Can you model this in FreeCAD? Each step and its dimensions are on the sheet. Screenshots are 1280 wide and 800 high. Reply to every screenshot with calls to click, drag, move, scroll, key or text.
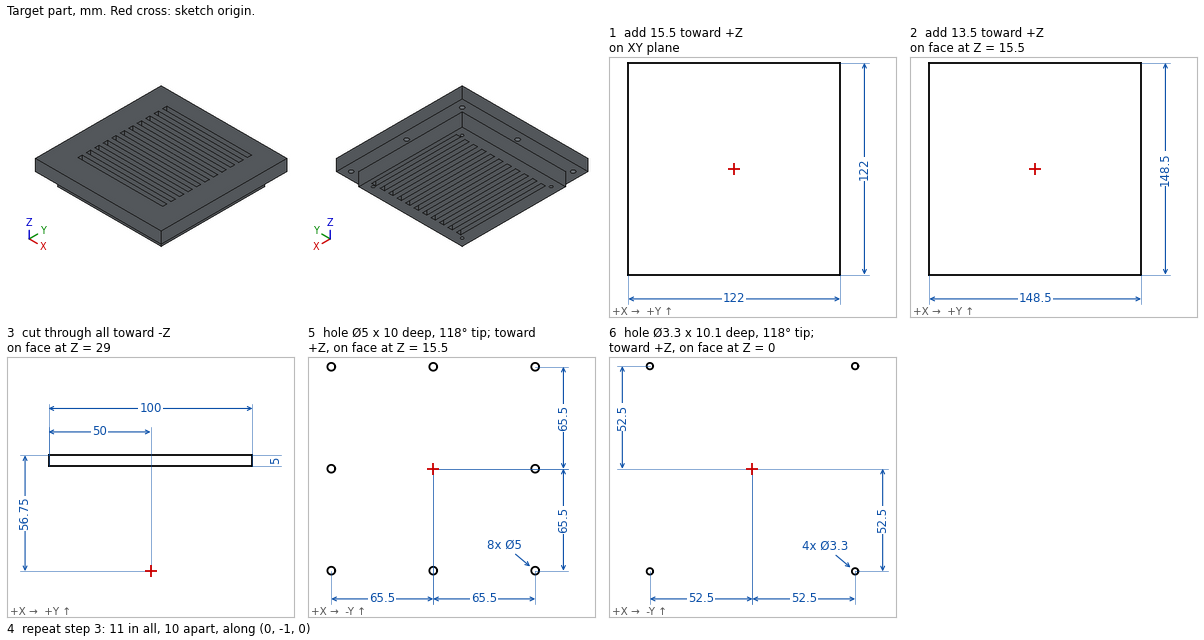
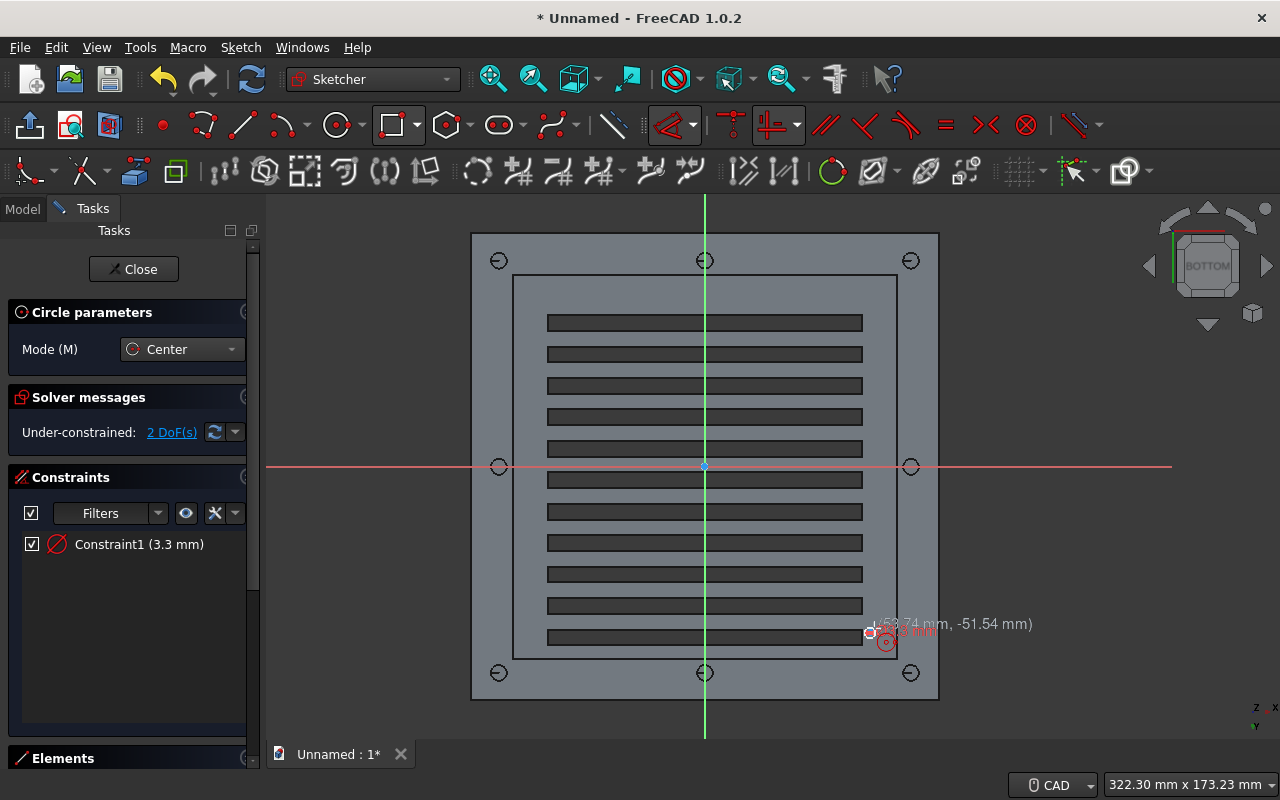
scroll(540, 632, up, 8)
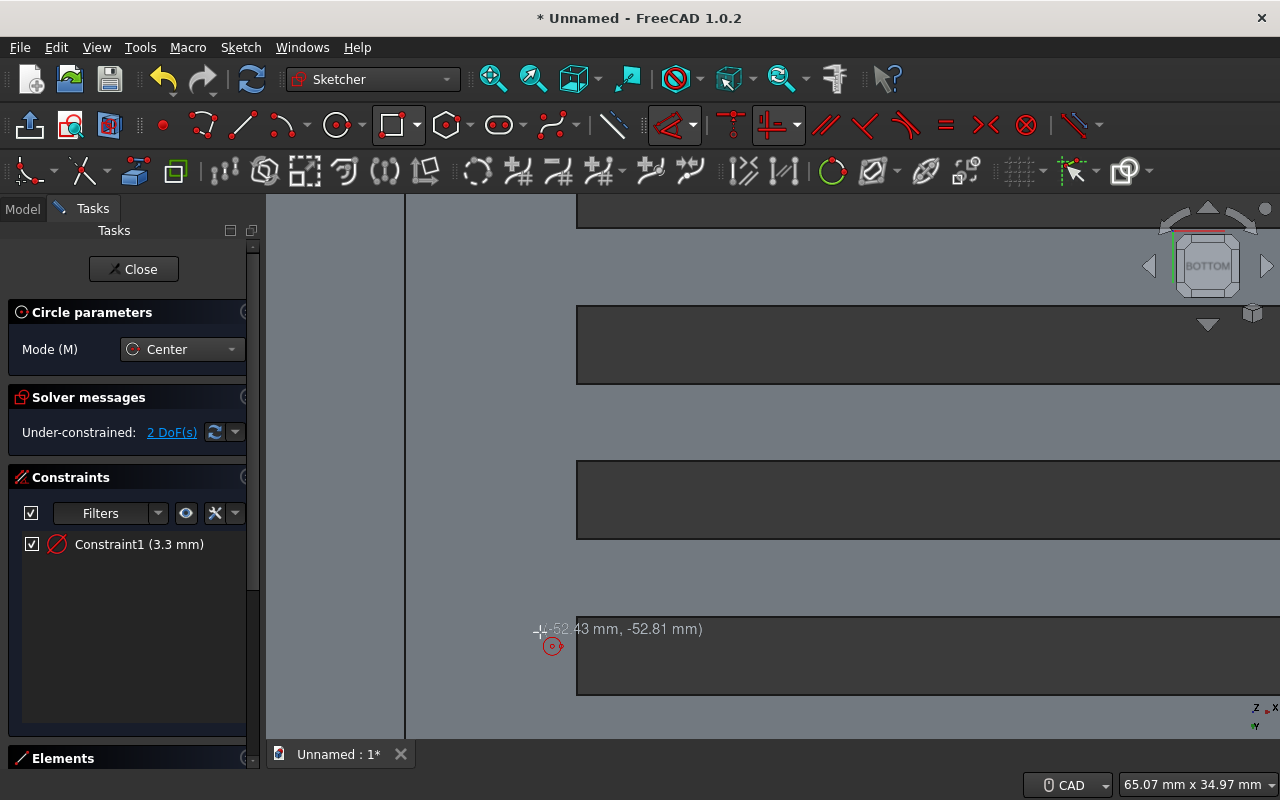
scroll(540, 632, down, 8)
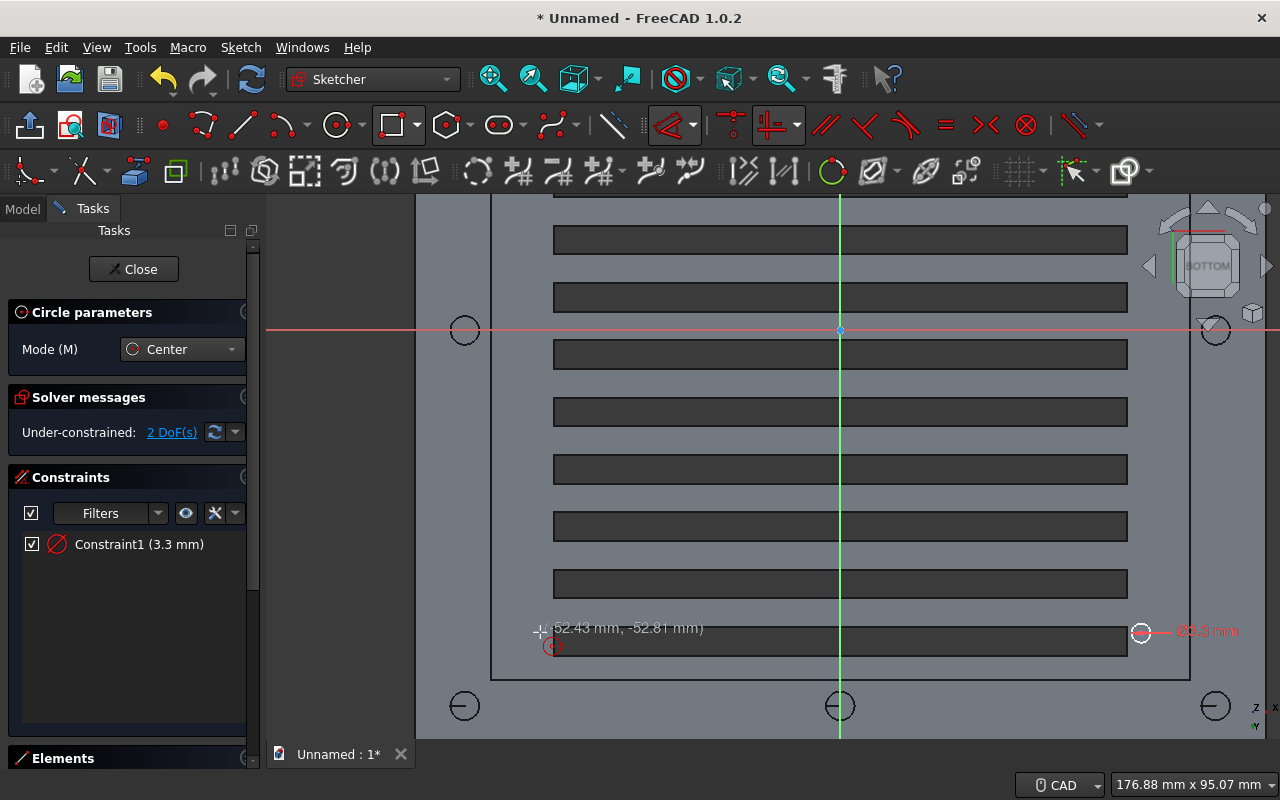
click(540, 632)
move(543, 628)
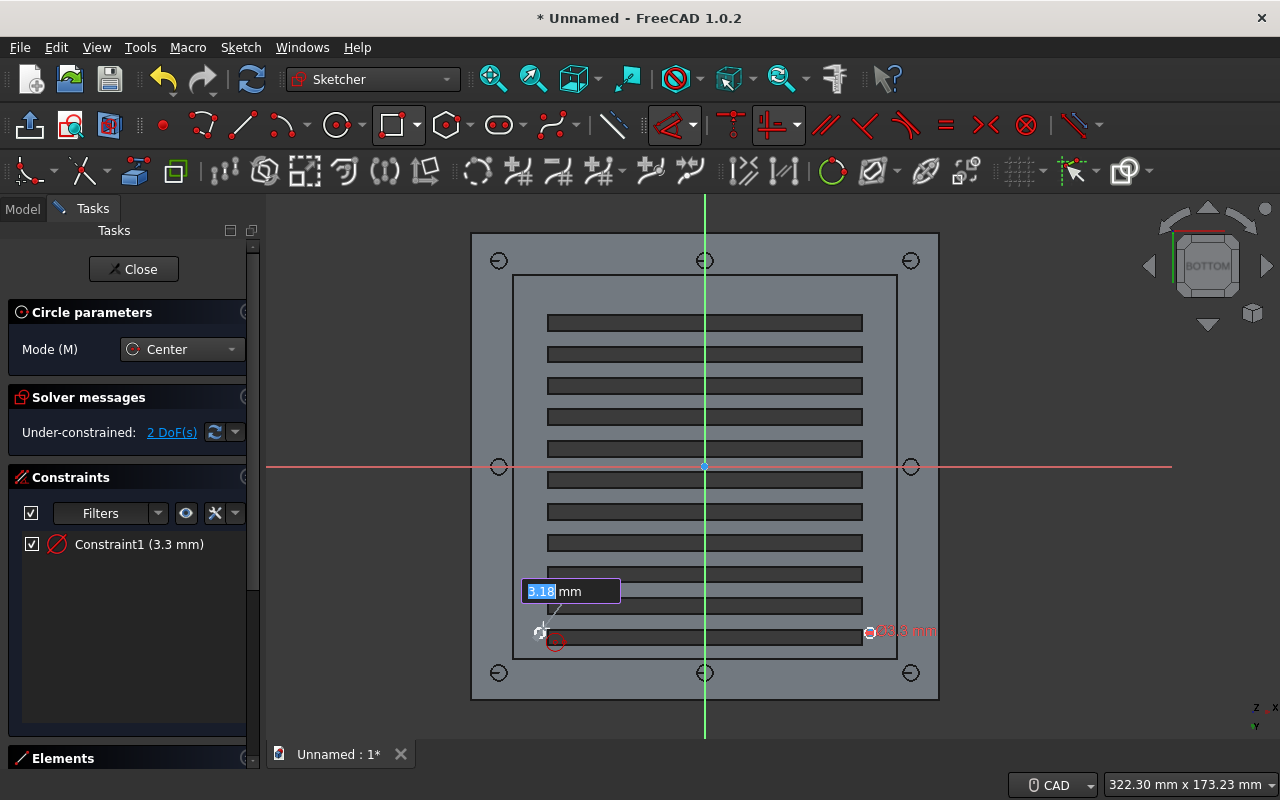
text(3.3)
key(Return)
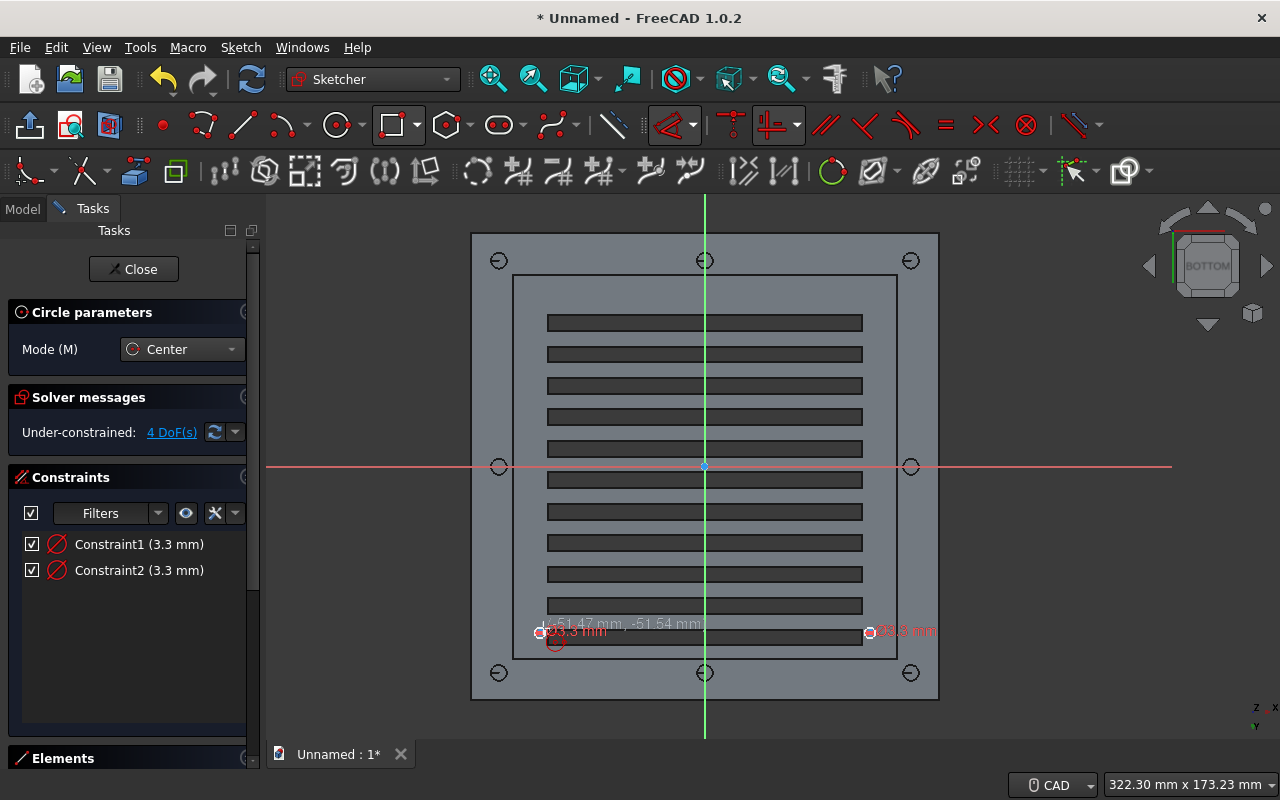
scroll(540, 302, up, 8)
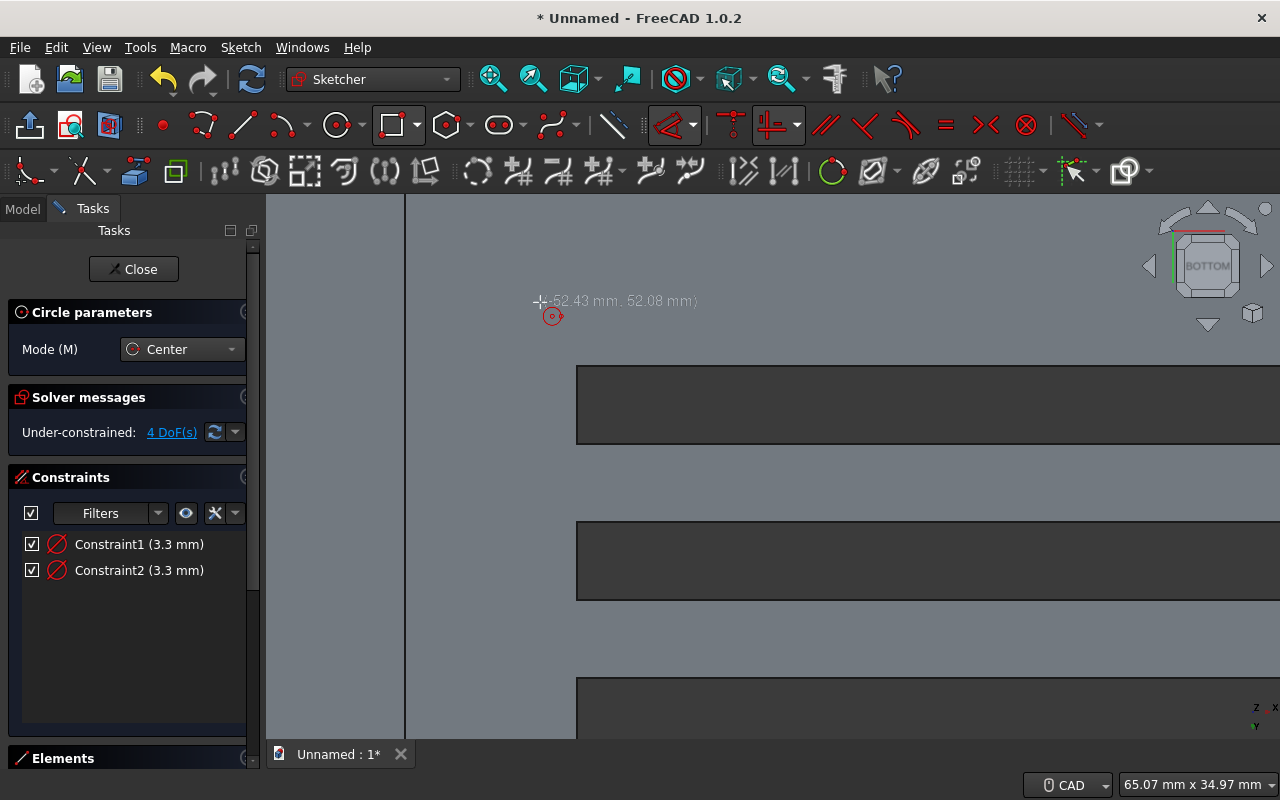
scroll(540, 302, down, 8)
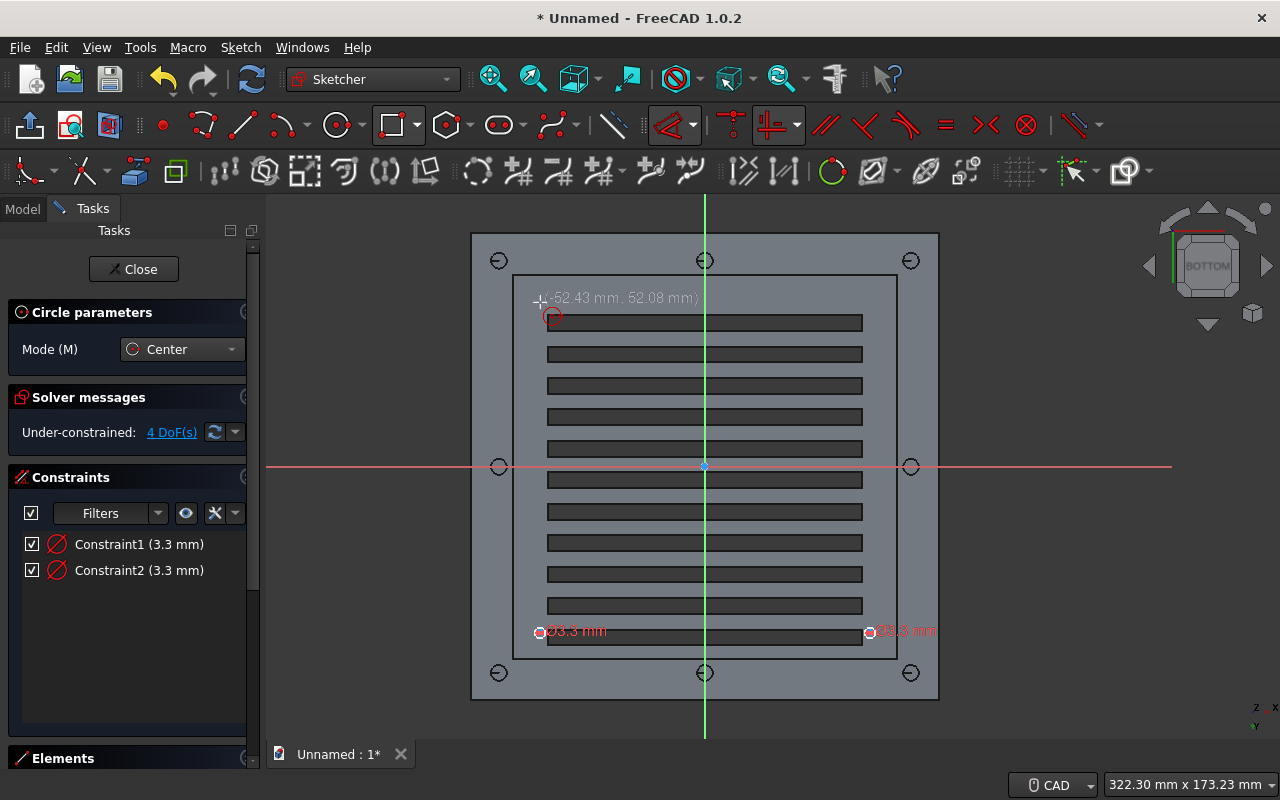
click(540, 302)
move(543, 298)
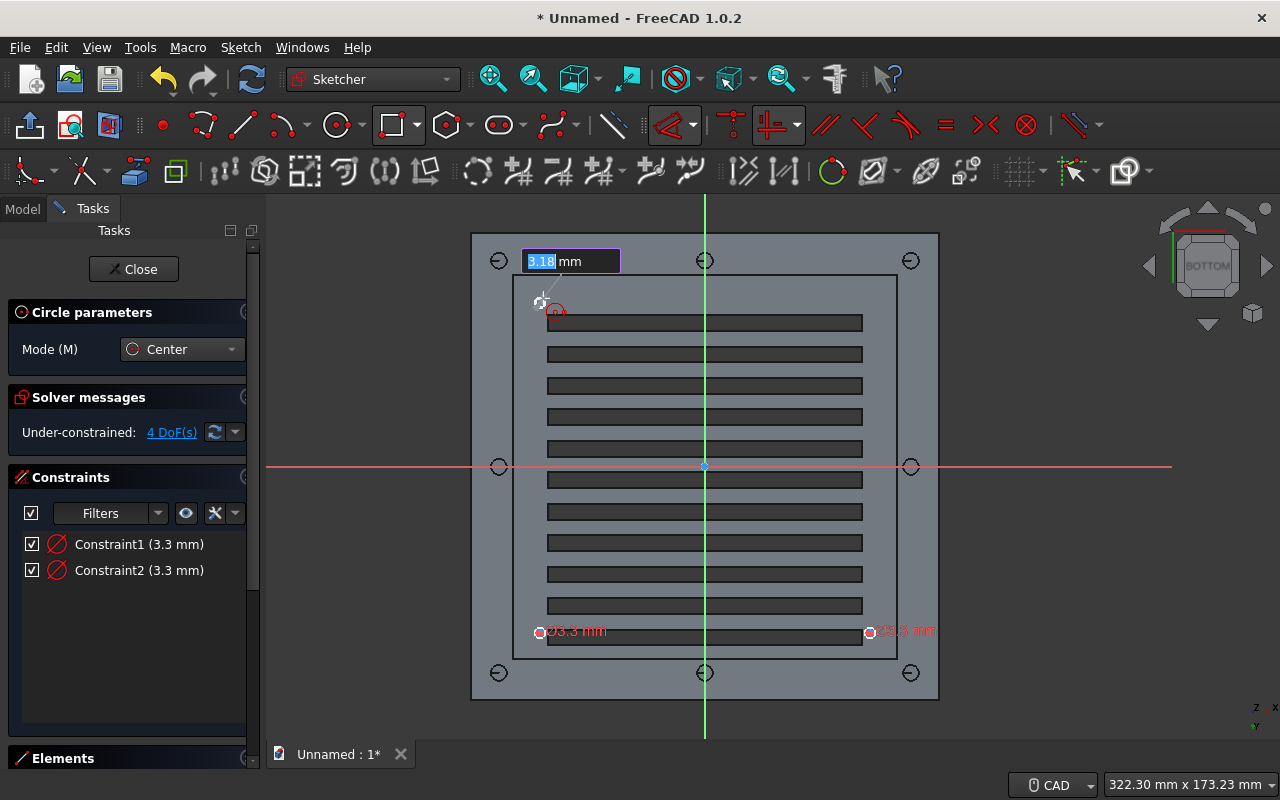
text(3.3)
key(Return)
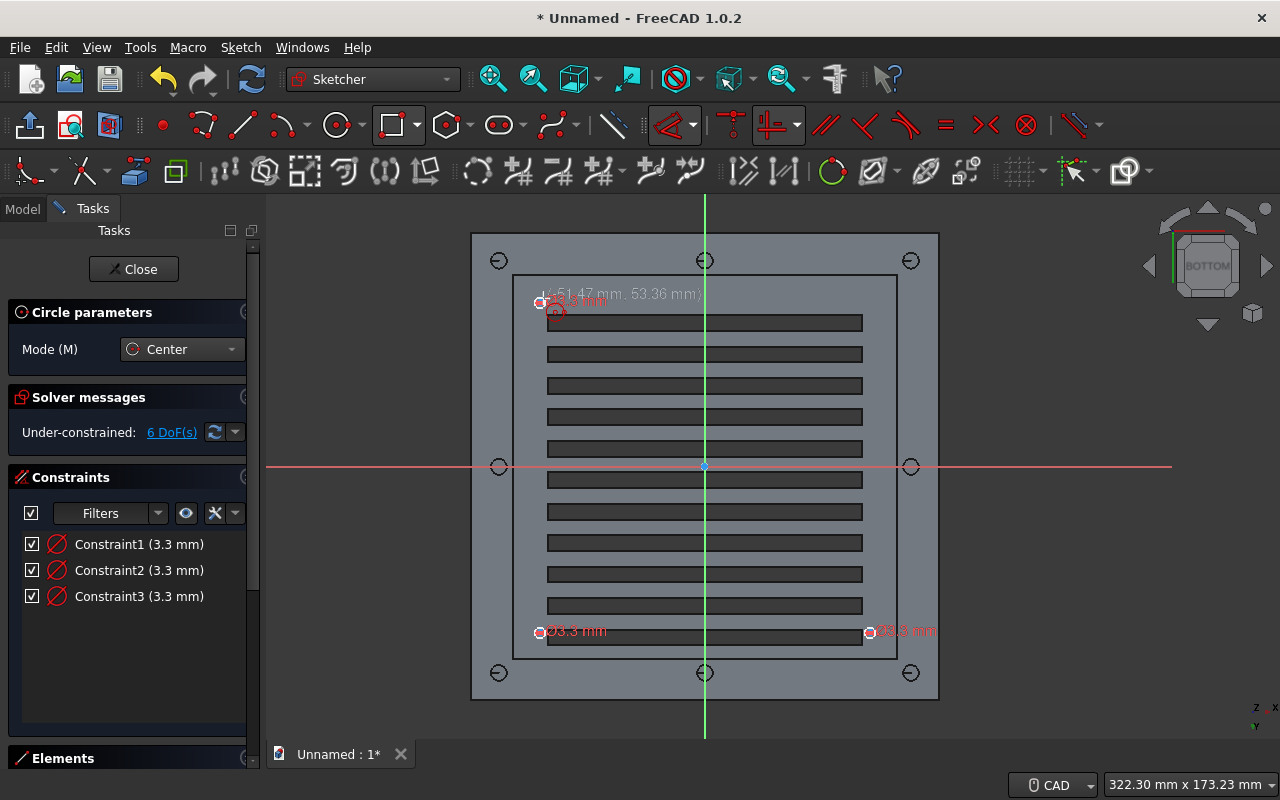
scroll(870, 302, up, 8)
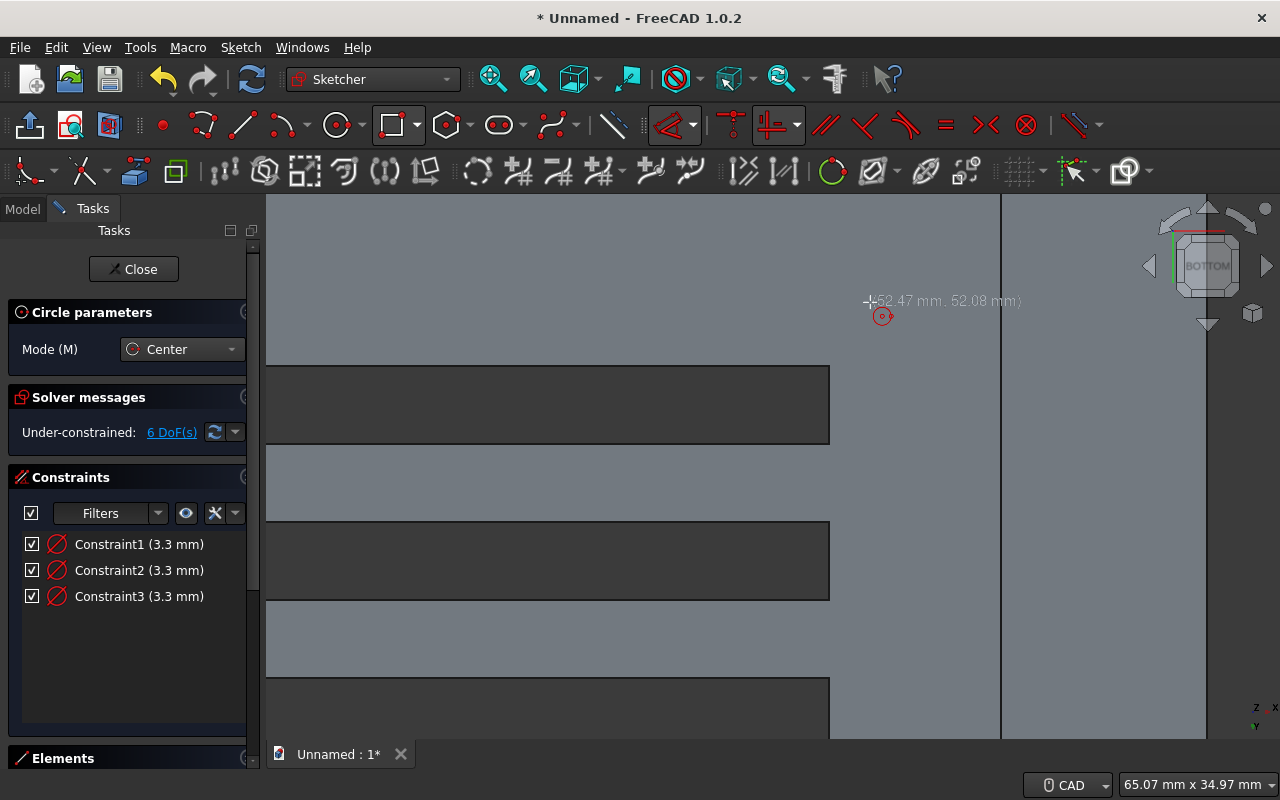
scroll(870, 302, down, 8)